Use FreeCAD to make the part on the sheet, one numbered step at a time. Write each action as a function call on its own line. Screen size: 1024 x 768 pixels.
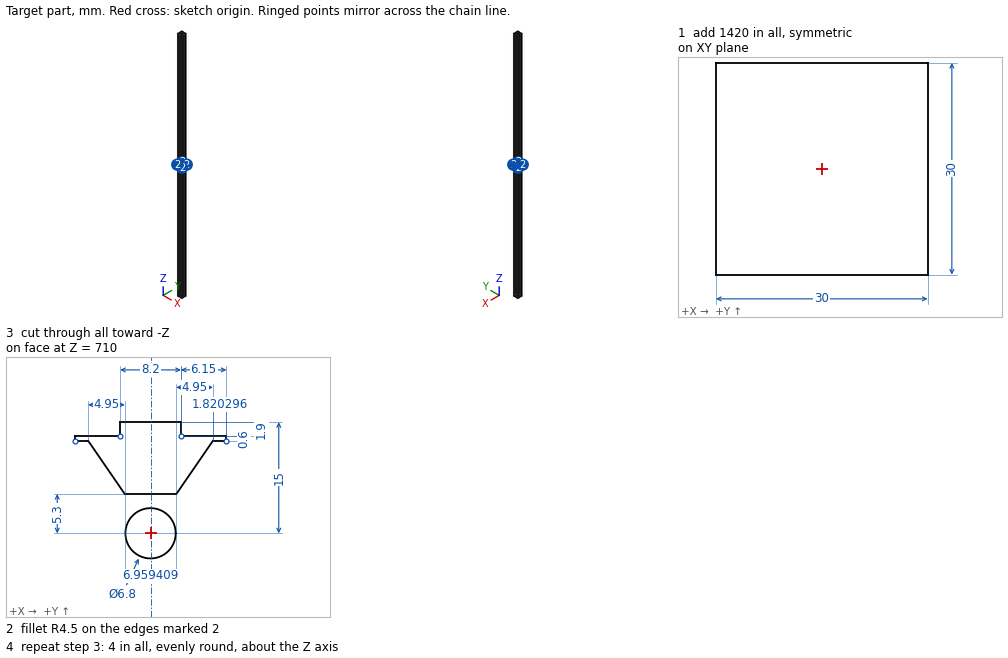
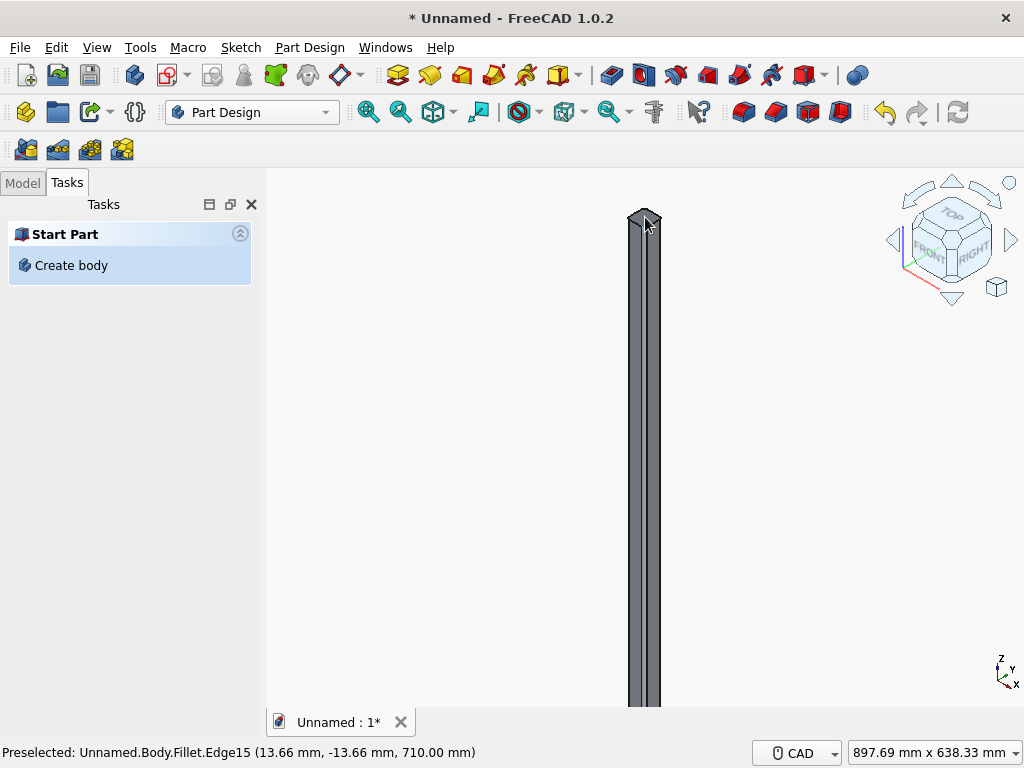
click(644, 214)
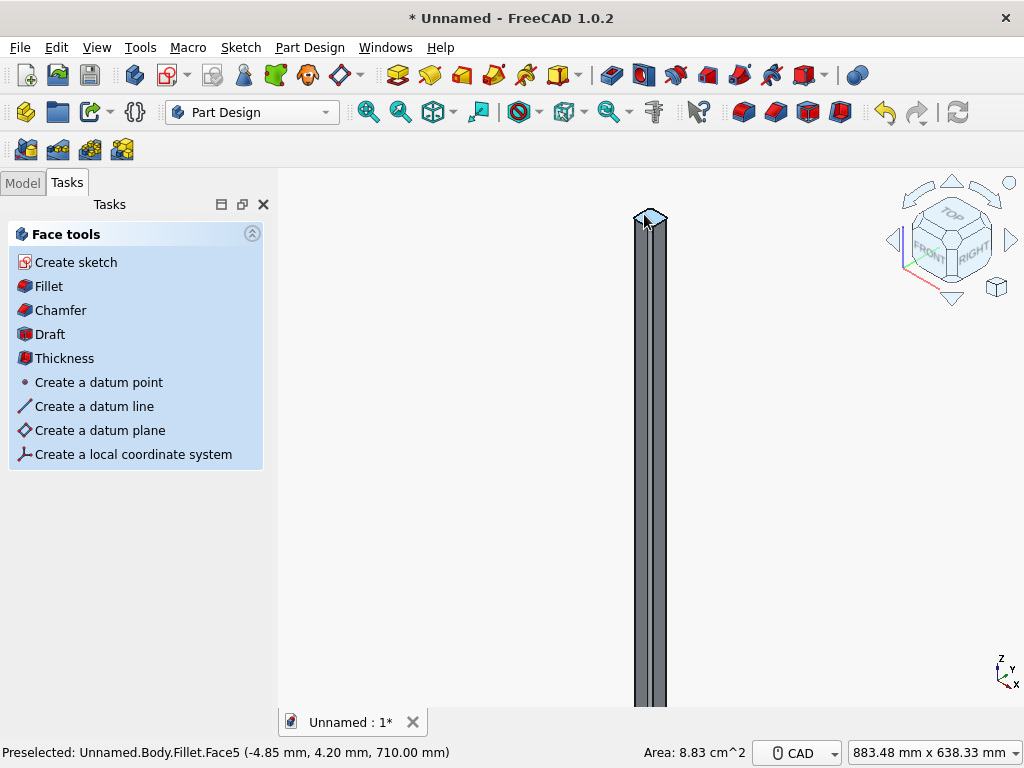
click(168, 76)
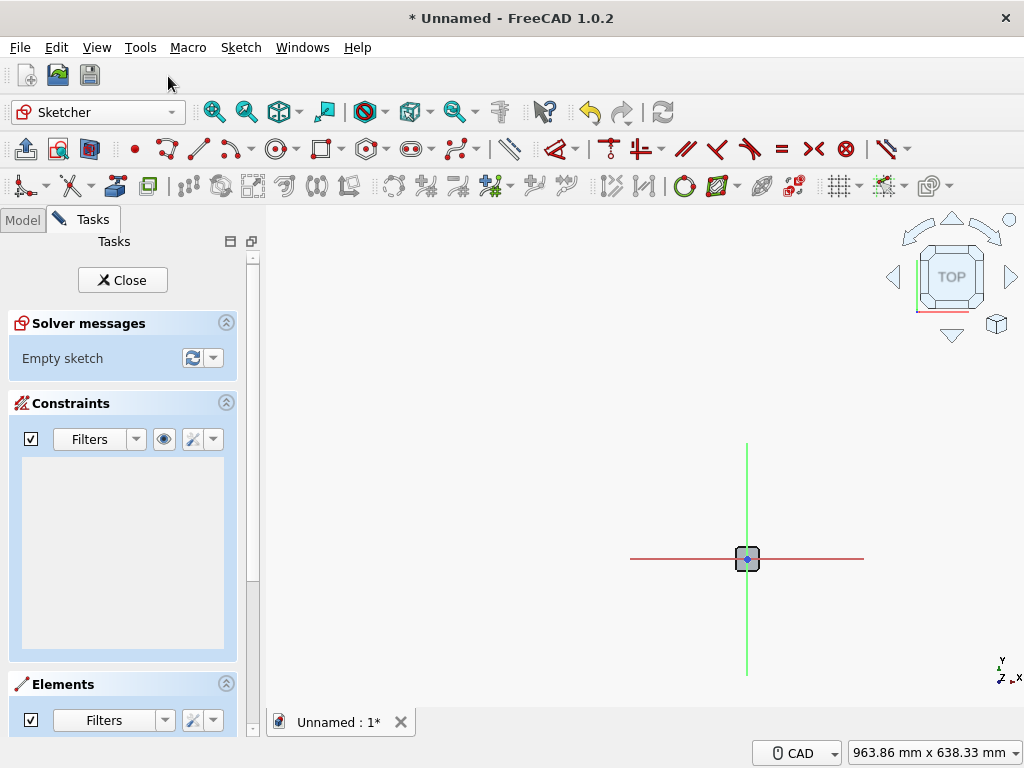
scroll(756, 560, up, 15)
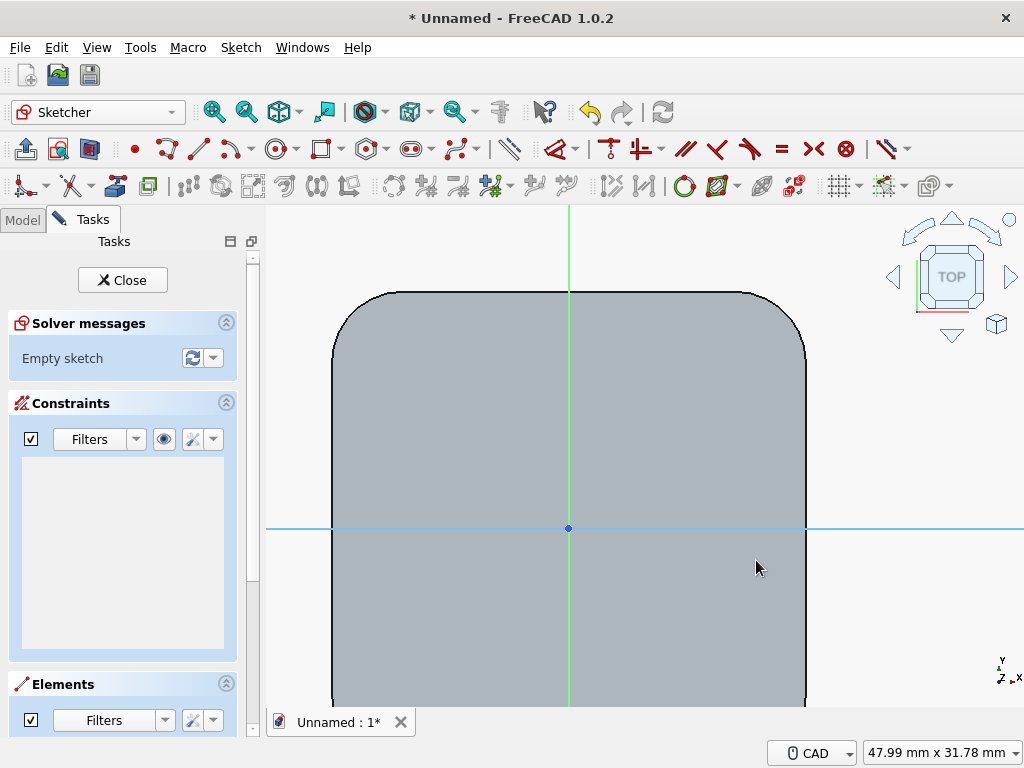
key(g)
key(m)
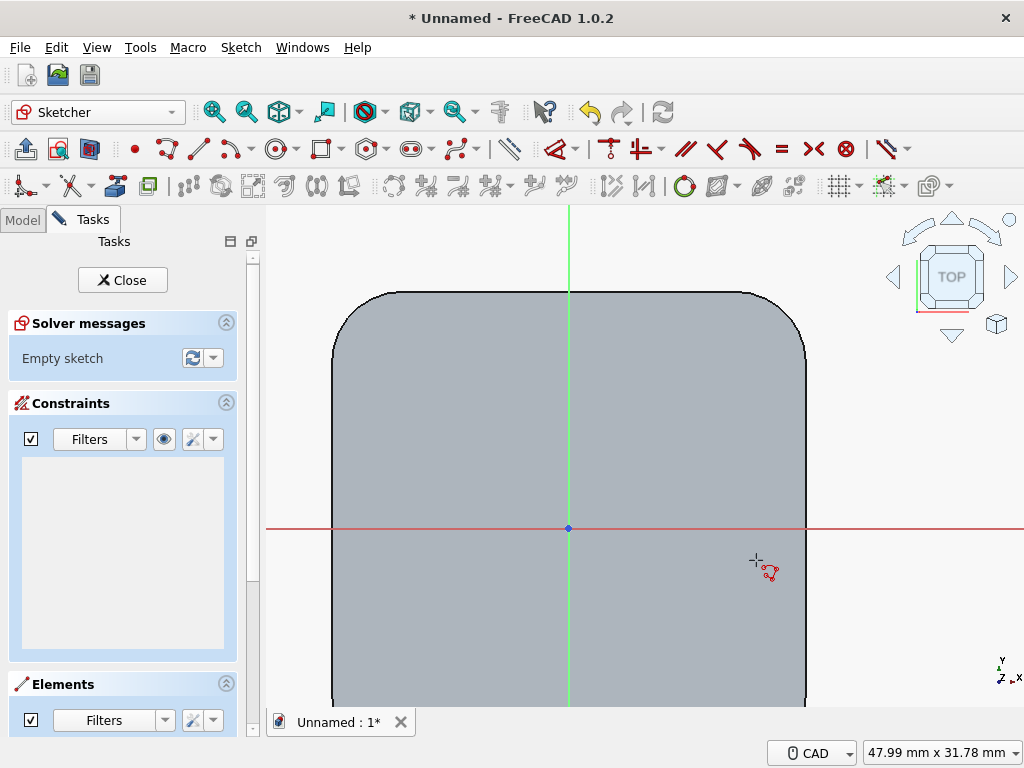
click(514, 445)
click(624, 445)
click(702, 331)
click(731, 331)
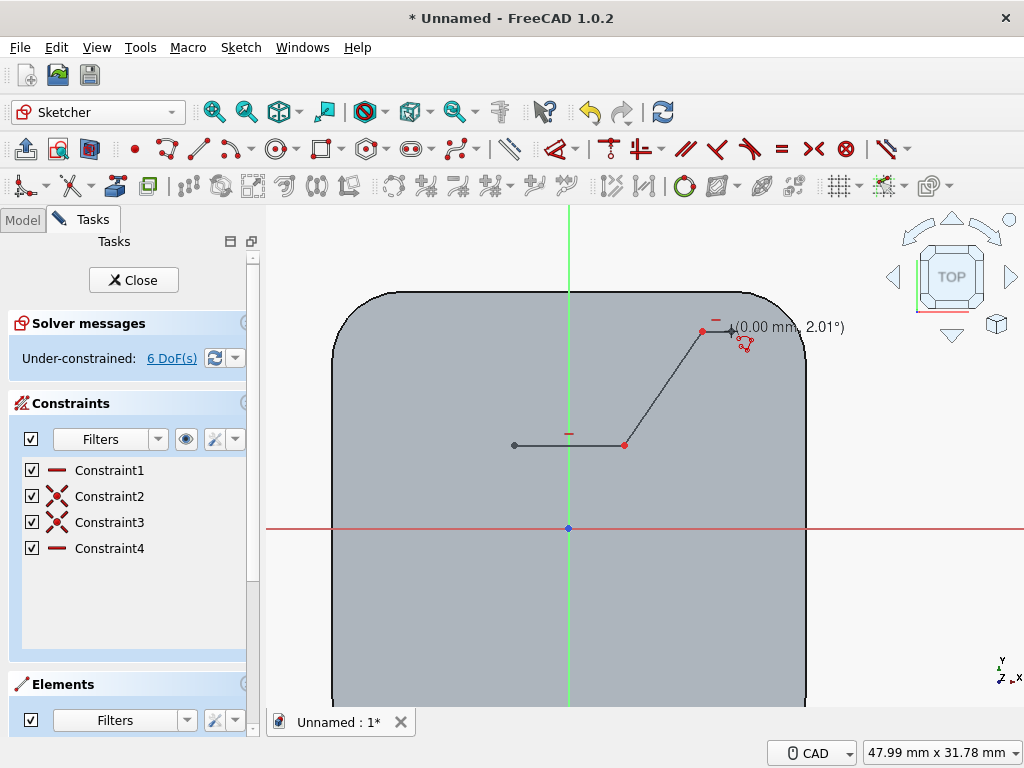
scroll(731, 322, up, 3)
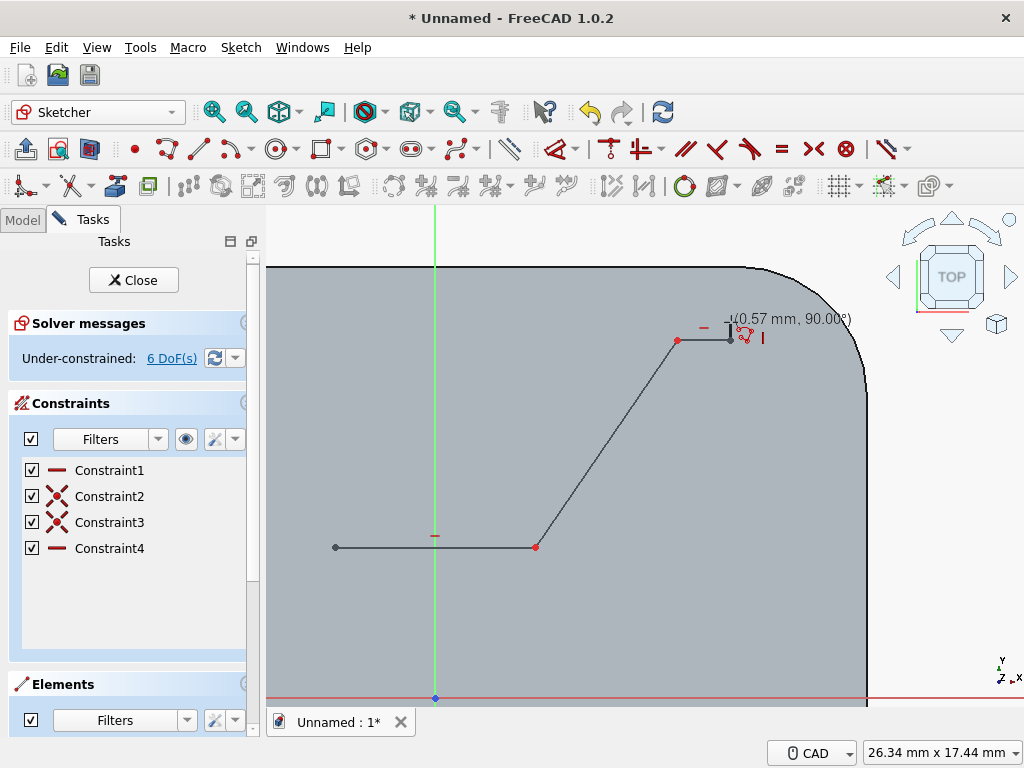
click(730, 321)
click(553, 321)
click(553, 267)
click(317, 267)
click(317, 321)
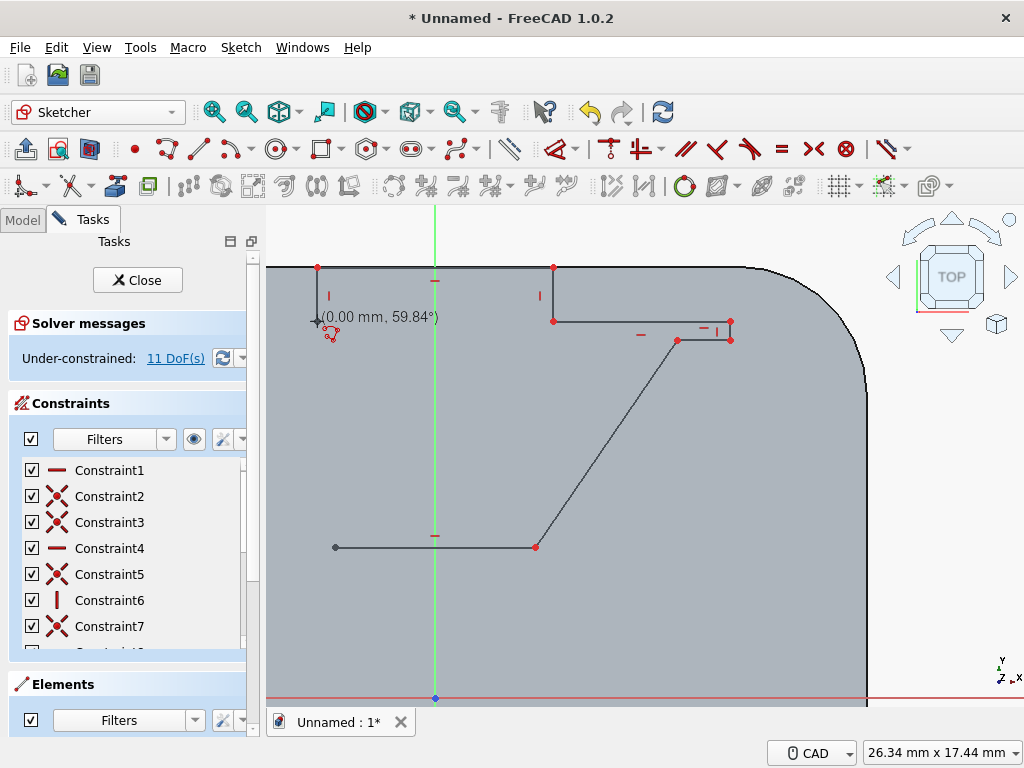
scroll(748, 364, down, 3)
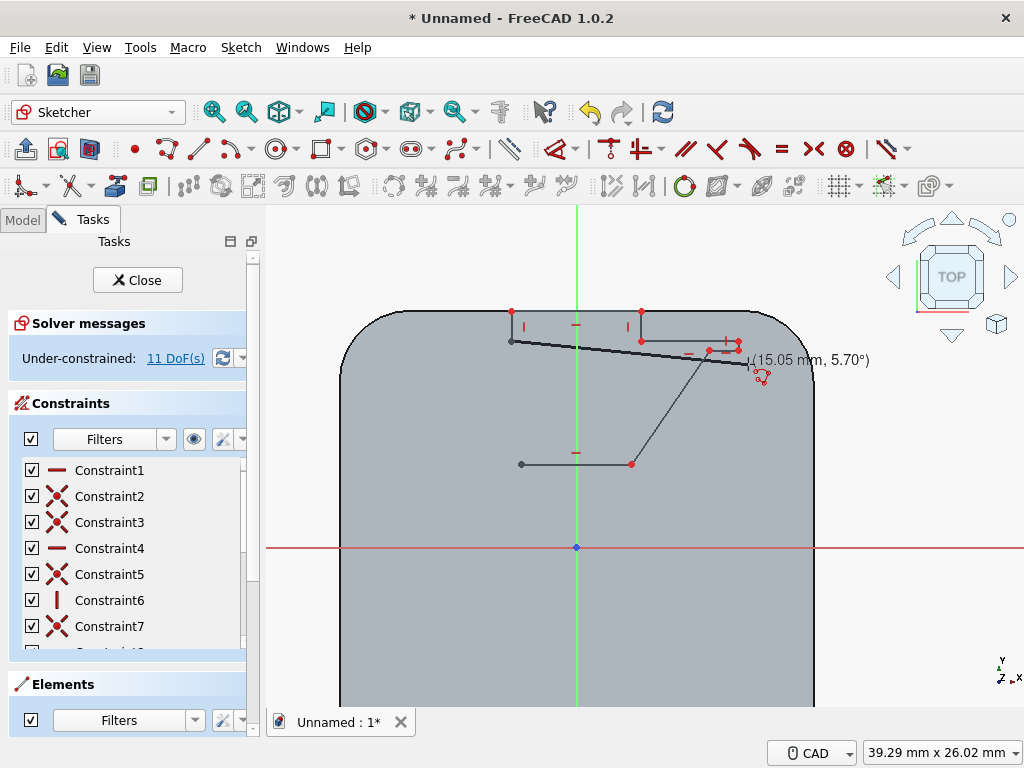
click(415, 341)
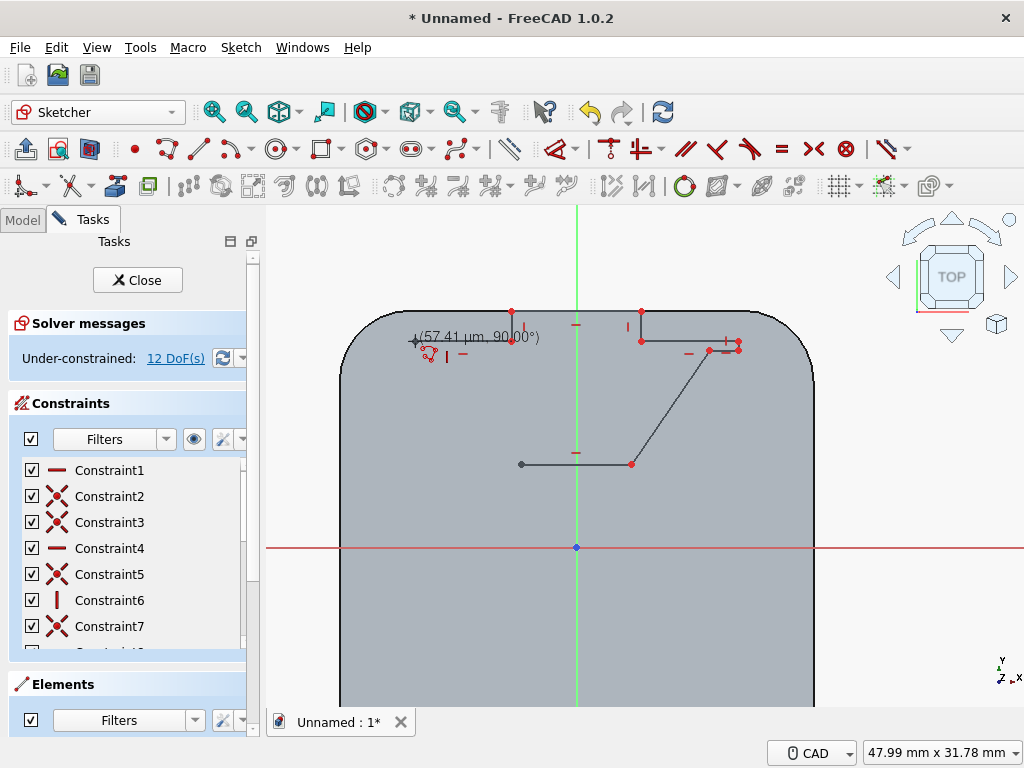
scroll(415, 350, up, 3)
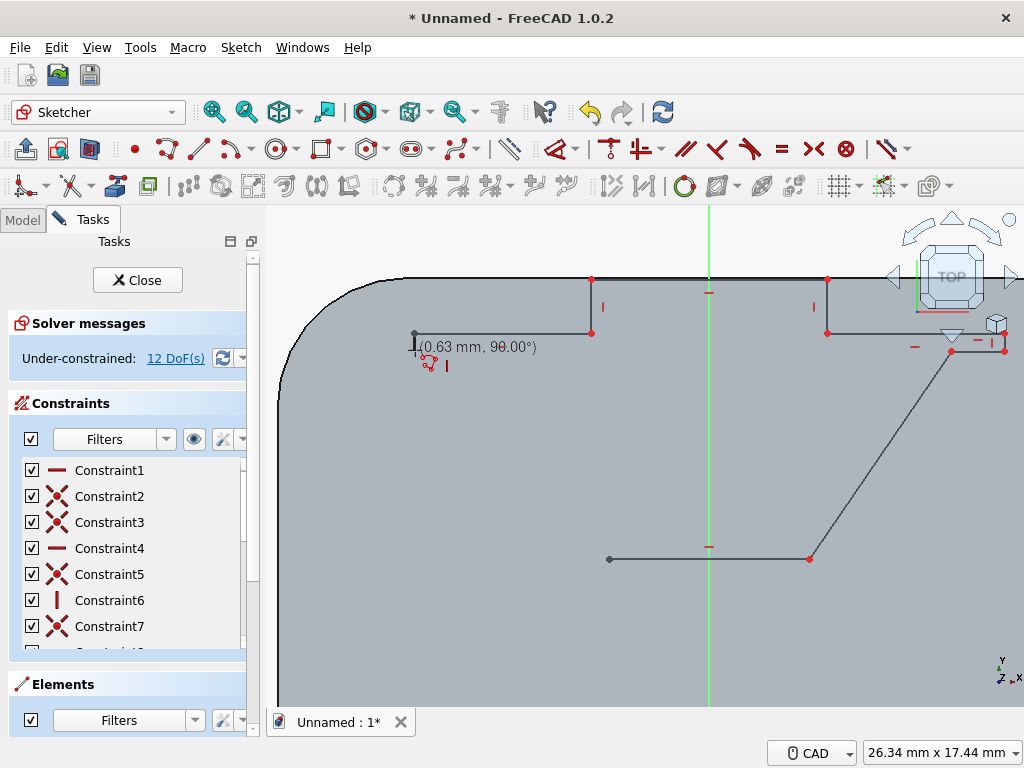
click(415, 350)
click(467, 350)
click(609, 559)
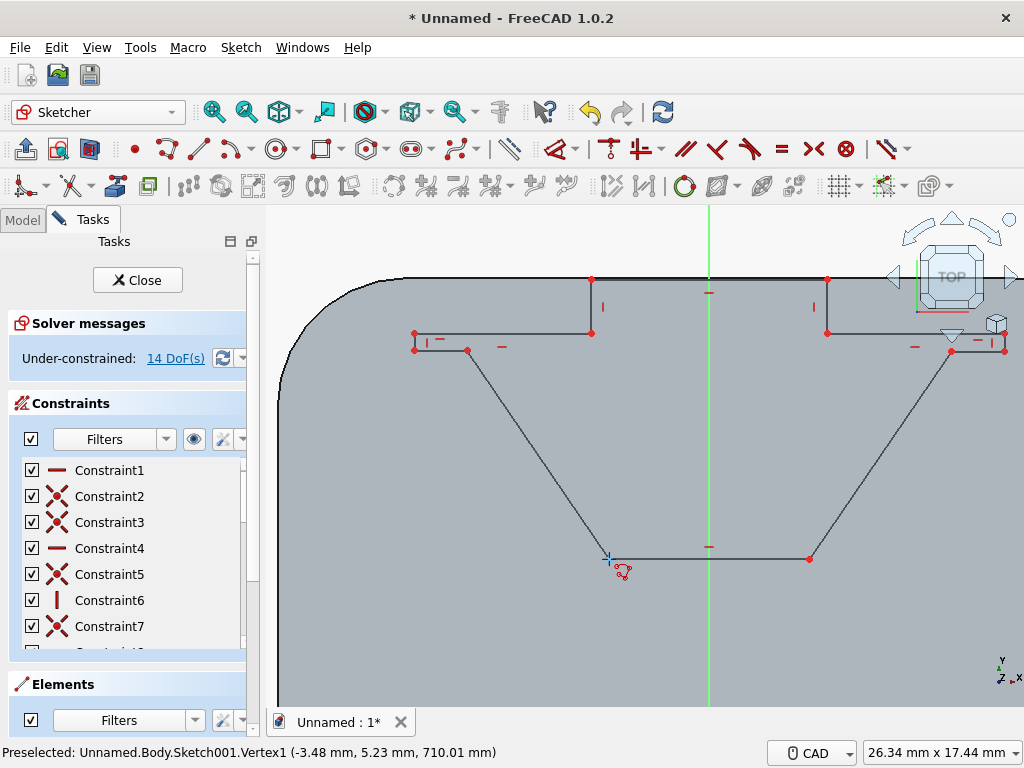
key(g)
key(c)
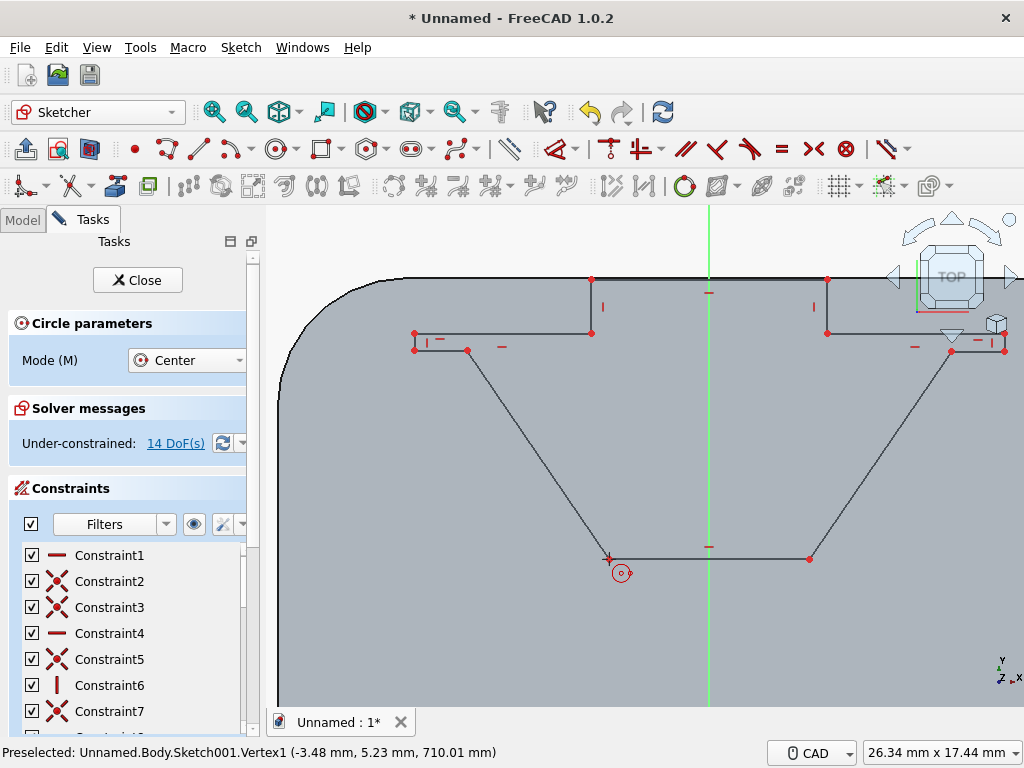
scroll(415, 350, down, 3)